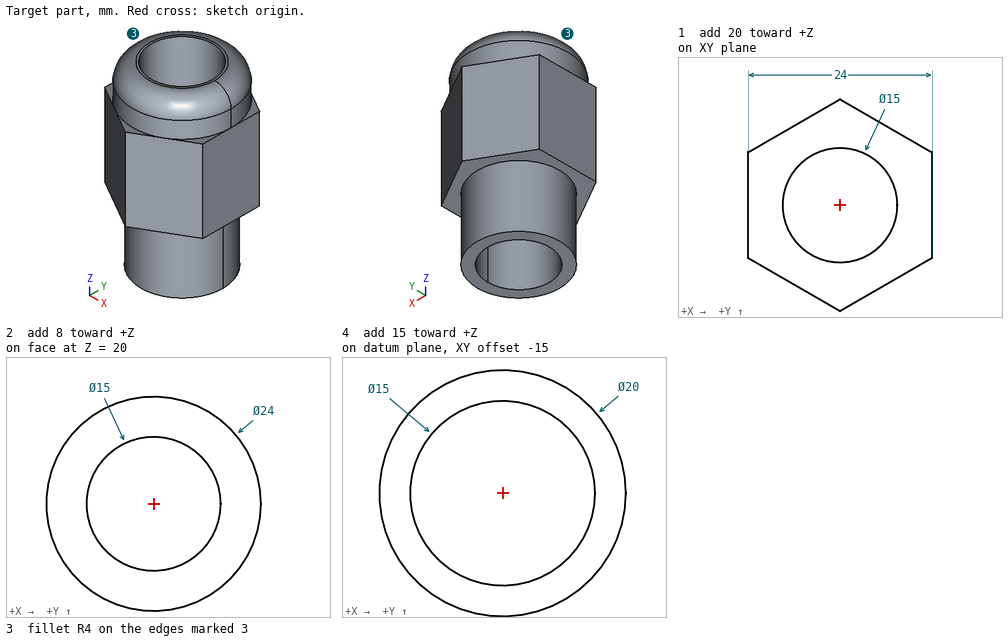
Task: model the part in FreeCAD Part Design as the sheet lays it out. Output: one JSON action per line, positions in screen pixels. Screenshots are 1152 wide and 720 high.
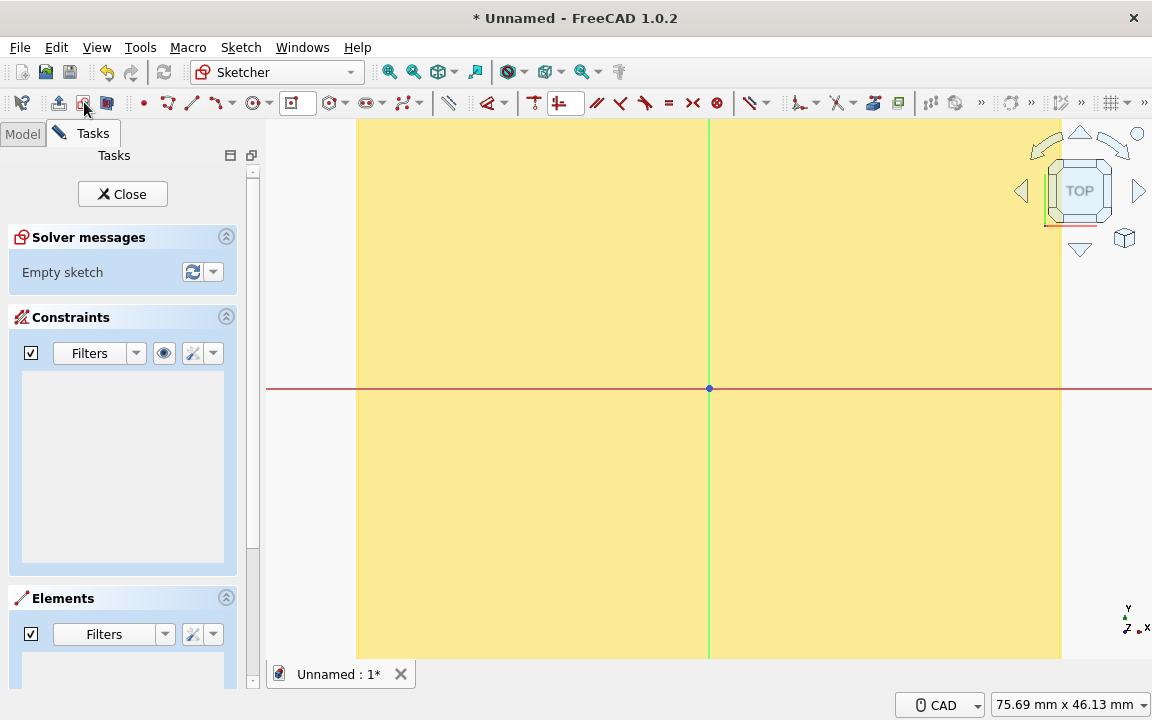
{"action": "scroll", "coordinate": [848, 389], "scroll_direction": "up", "scroll_amount": 2}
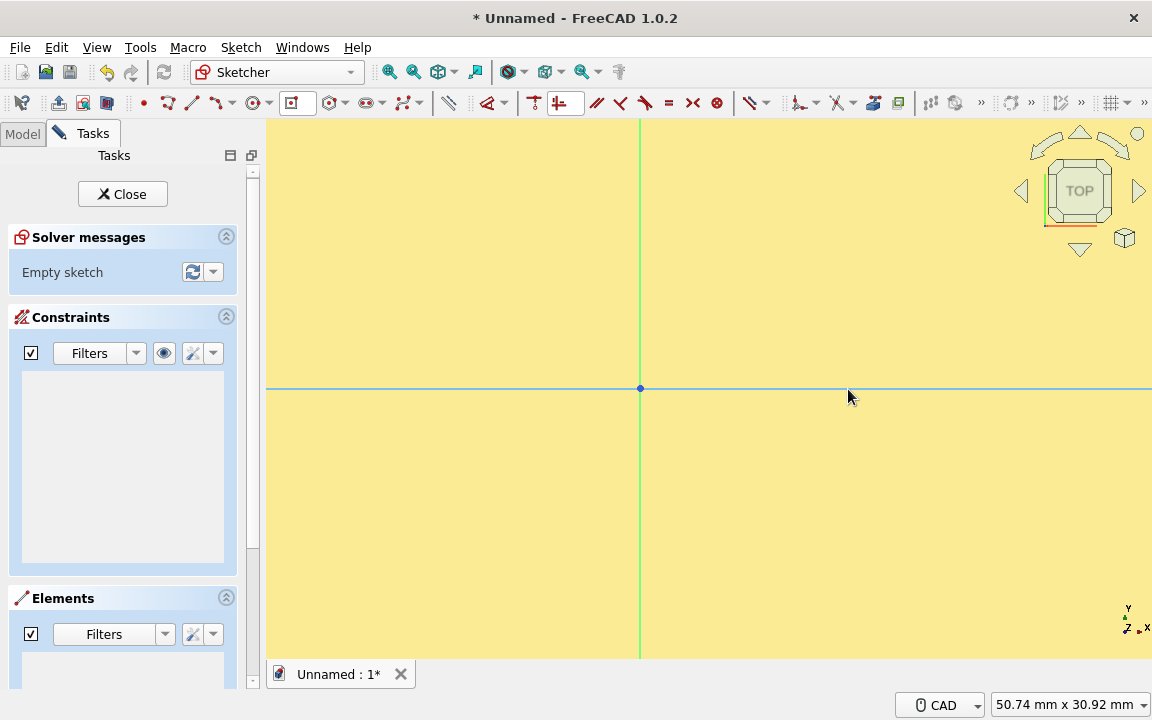
{"action": "key", "text": "g c"}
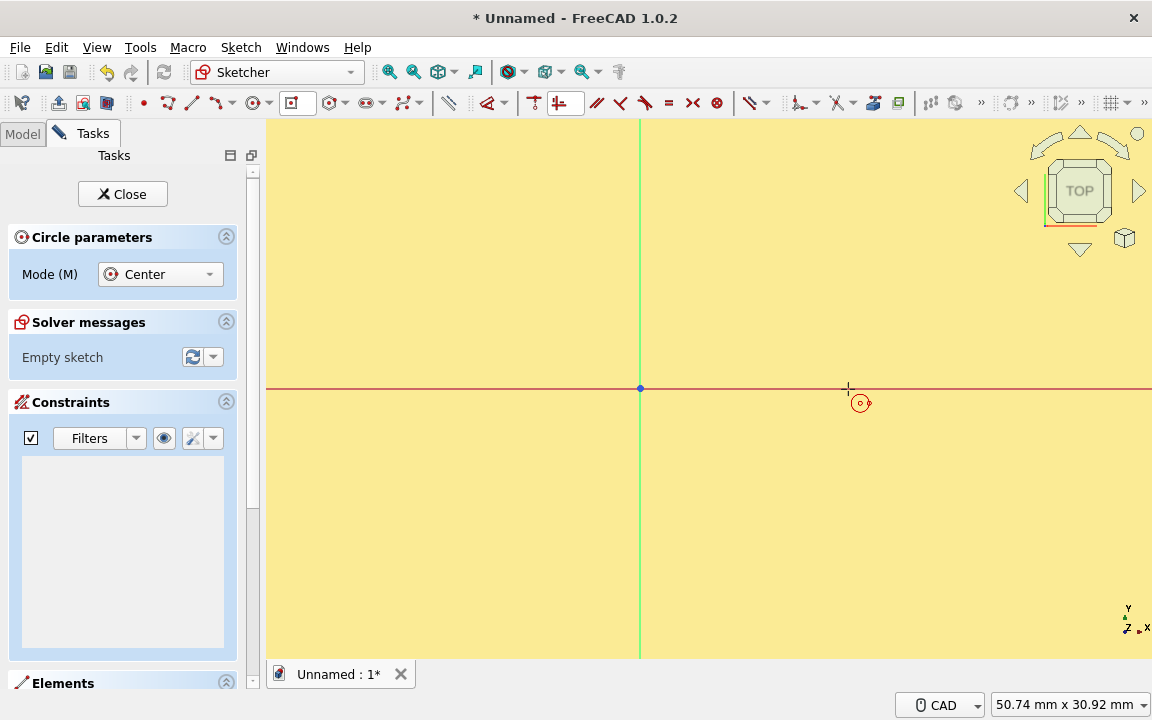
{"action": "left_click", "coordinate": [640, 389]}
{"action": "mouse_move", "coordinate": [764, 265]}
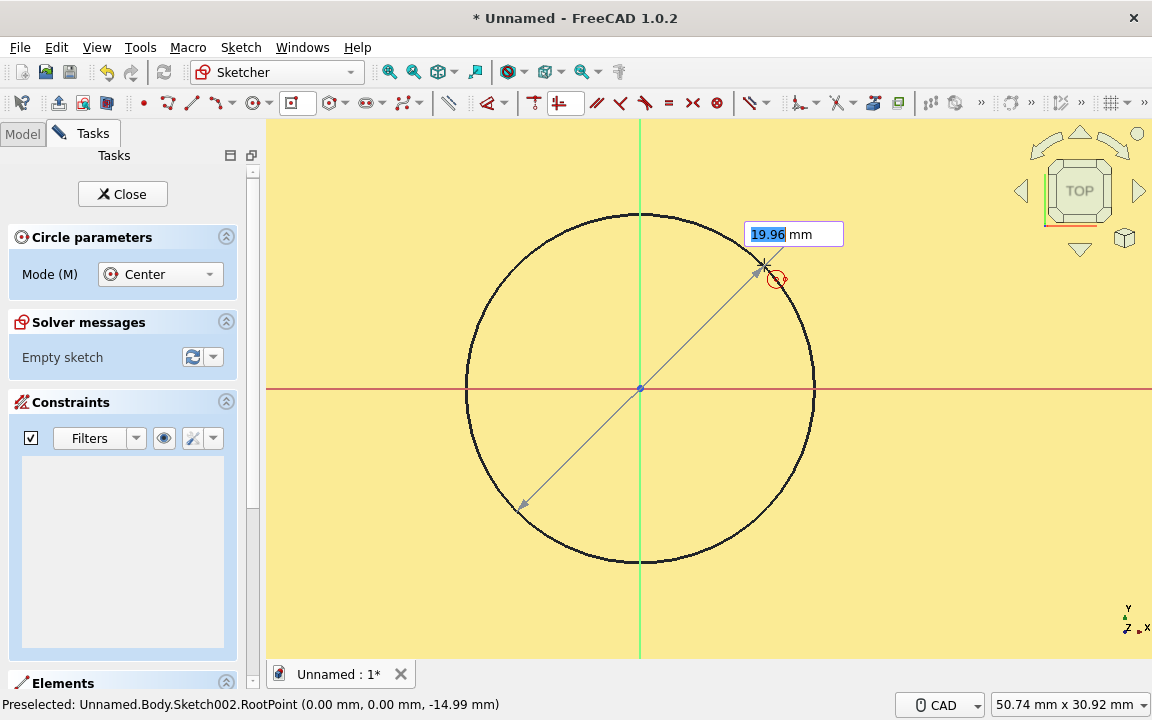
{"action": "type", "text": "20"}
{"action": "key", "text": "Return"}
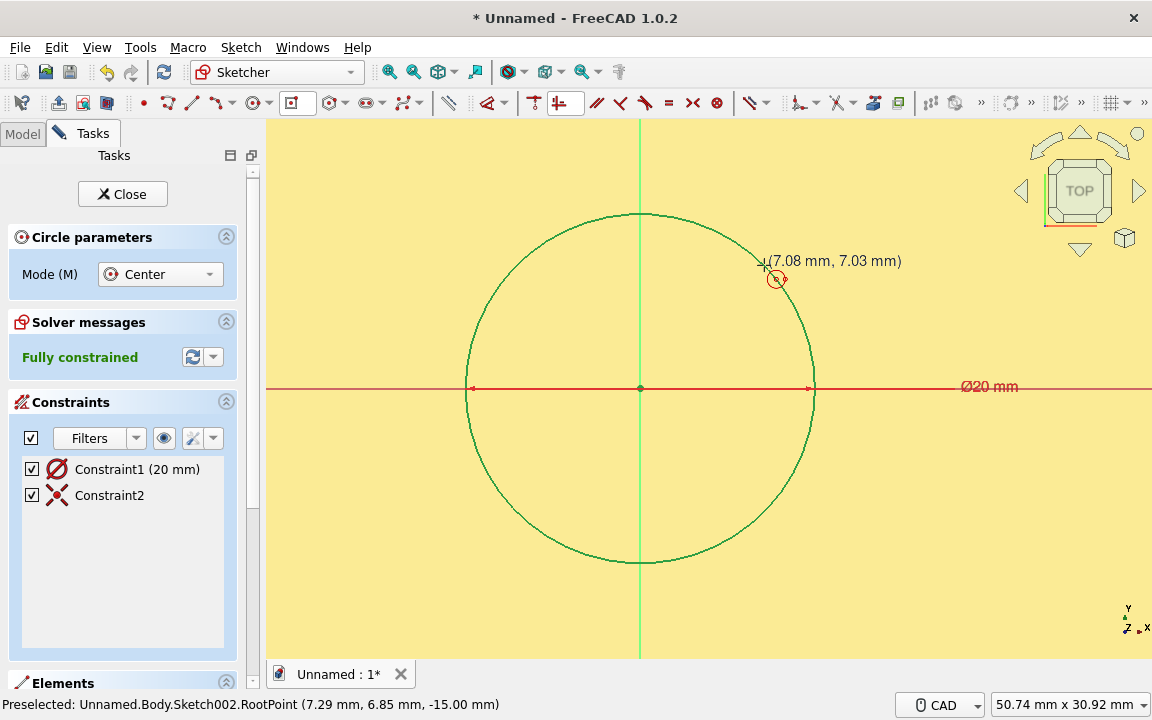
{"action": "left_click", "coordinate": [640, 389]}
{"action": "mouse_move", "coordinate": [733, 296]}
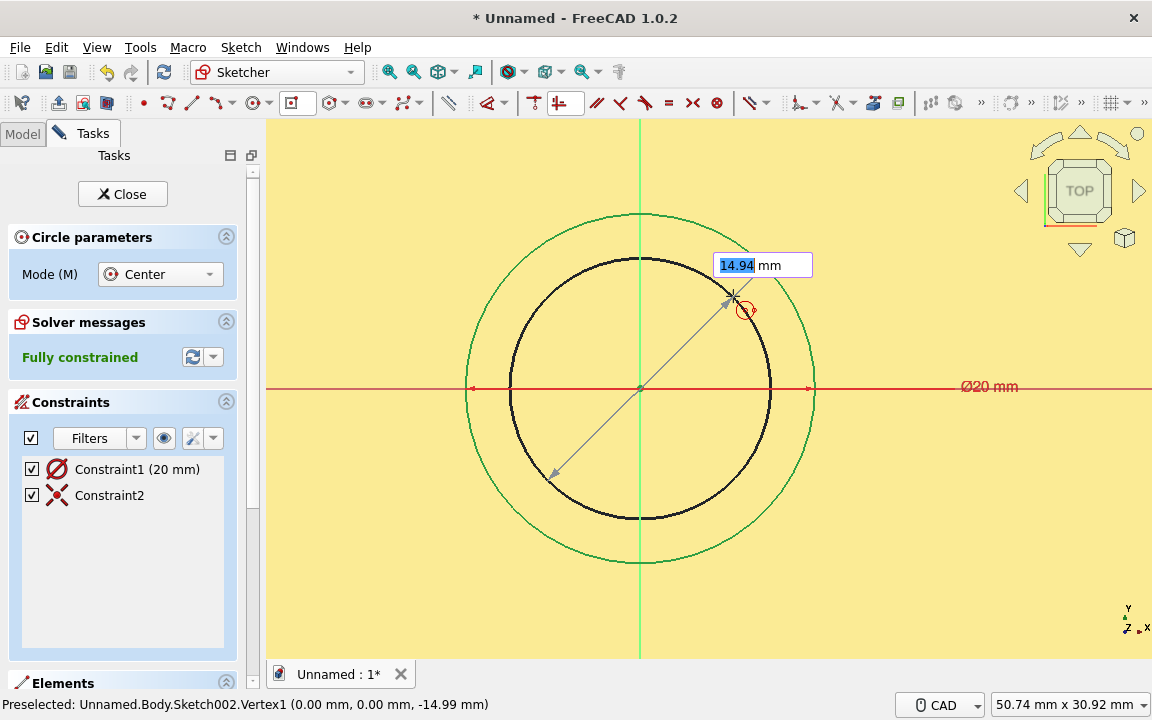
{"action": "type", "text": "15"}
{"action": "key", "text": "Return"}
{"action": "key", "text": "Escape"}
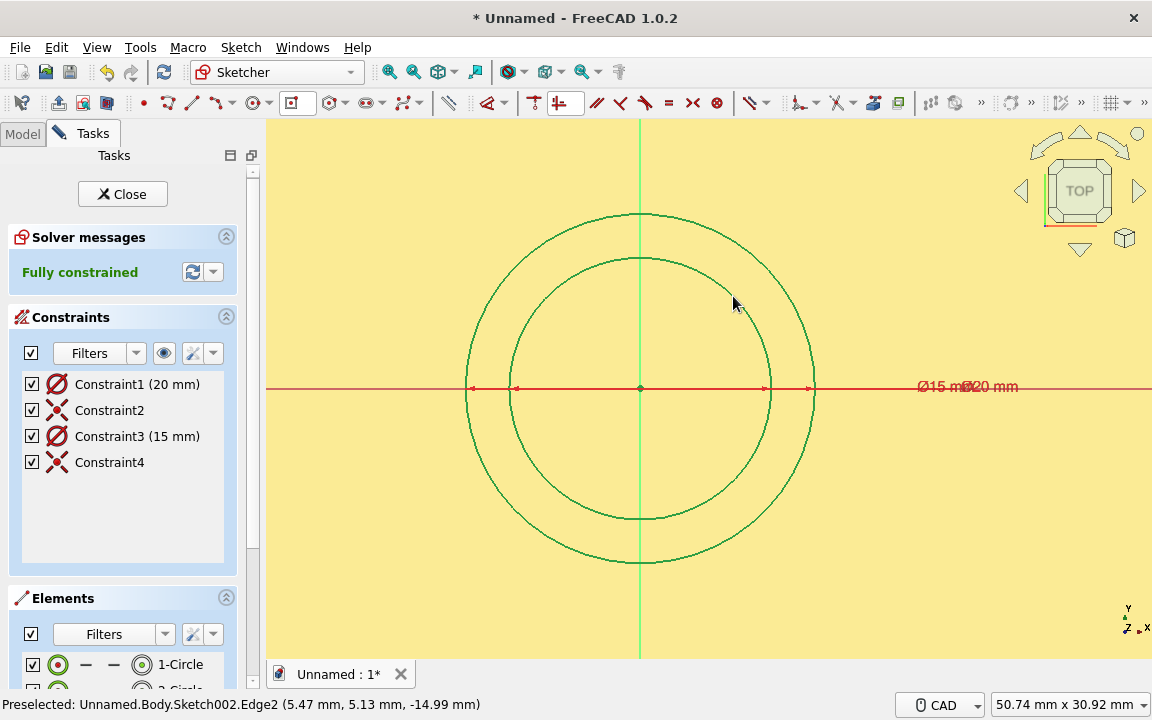
{"action": "left_click", "coordinate": [123, 194]}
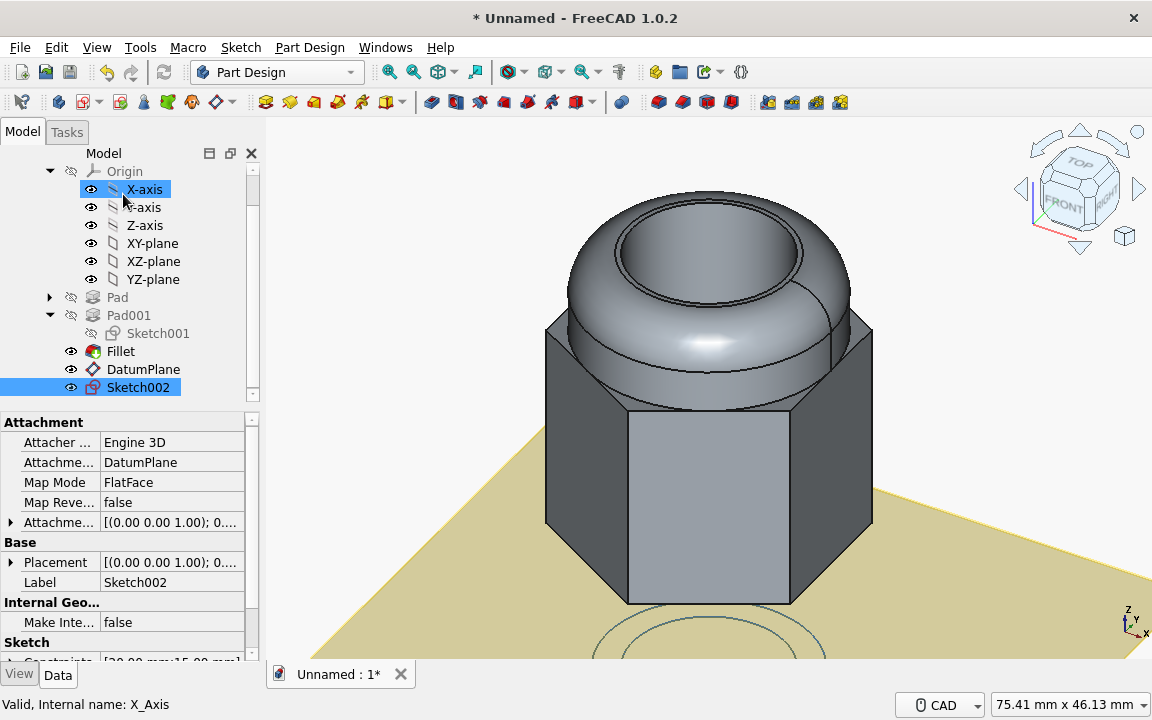
{"action": "left_click", "coordinate": [266, 102]}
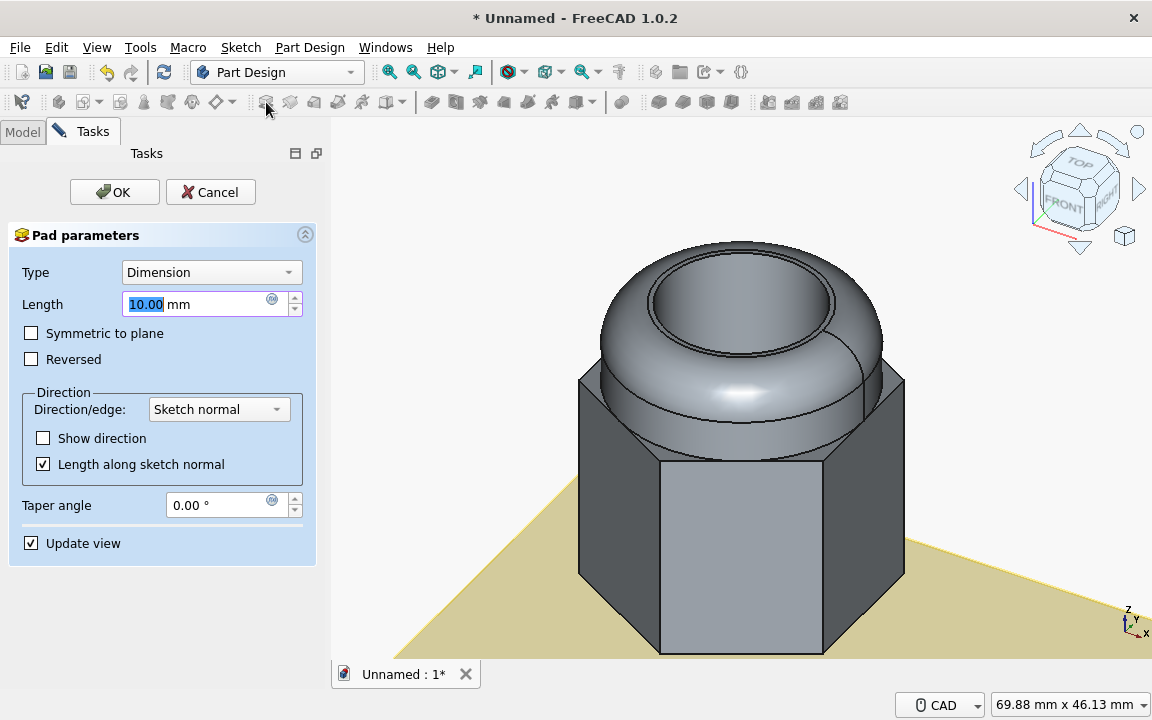
{"action": "type", "text": "15"}
{"action": "key", "text": "Tab"}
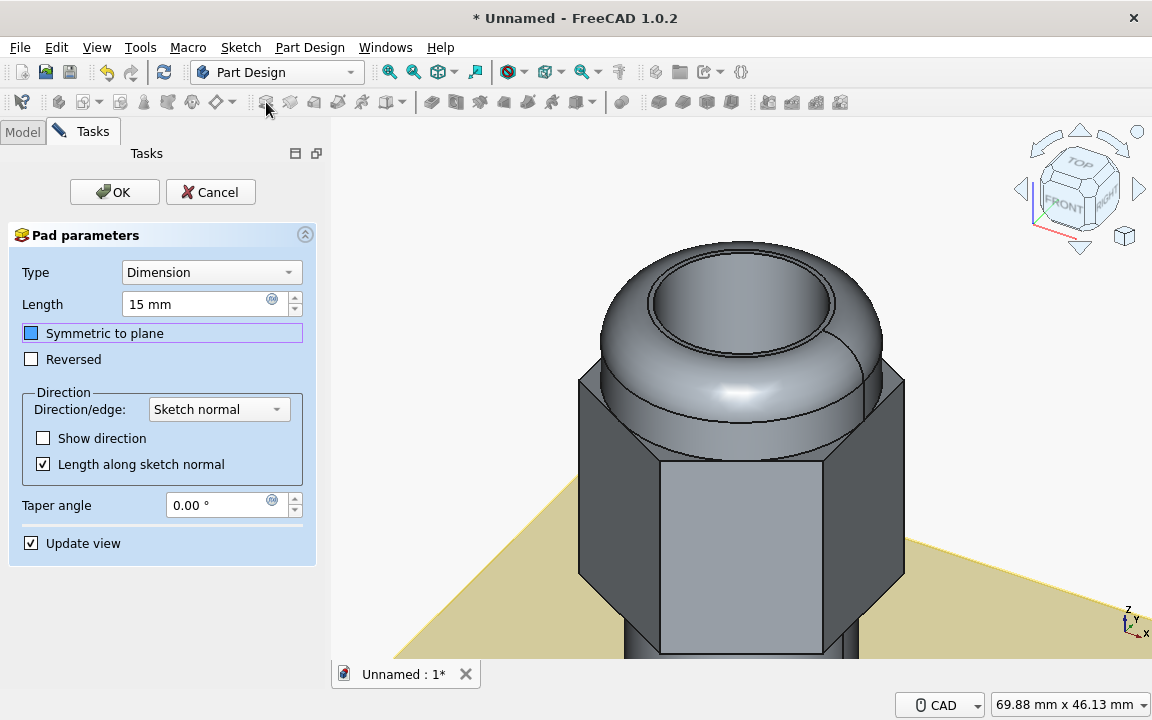
{"action": "left_click", "coordinate": [115, 192]}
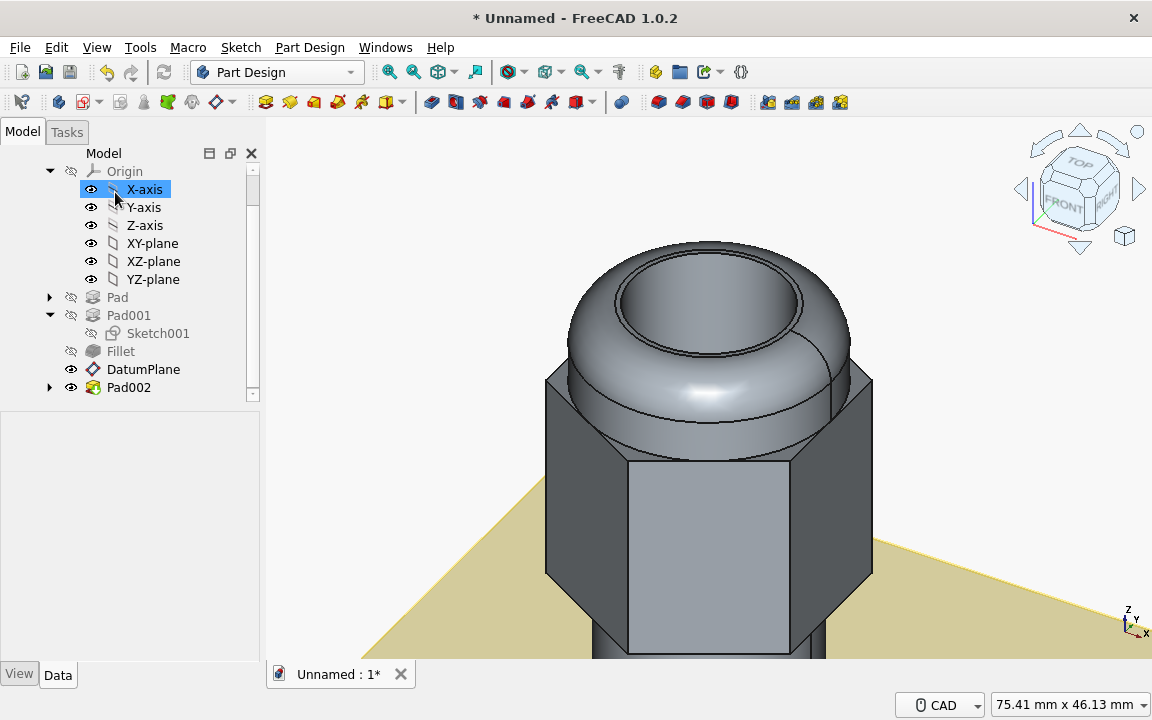
{"action": "left_click", "coordinate": [116, 369]}
{"action": "key", "text": "space"}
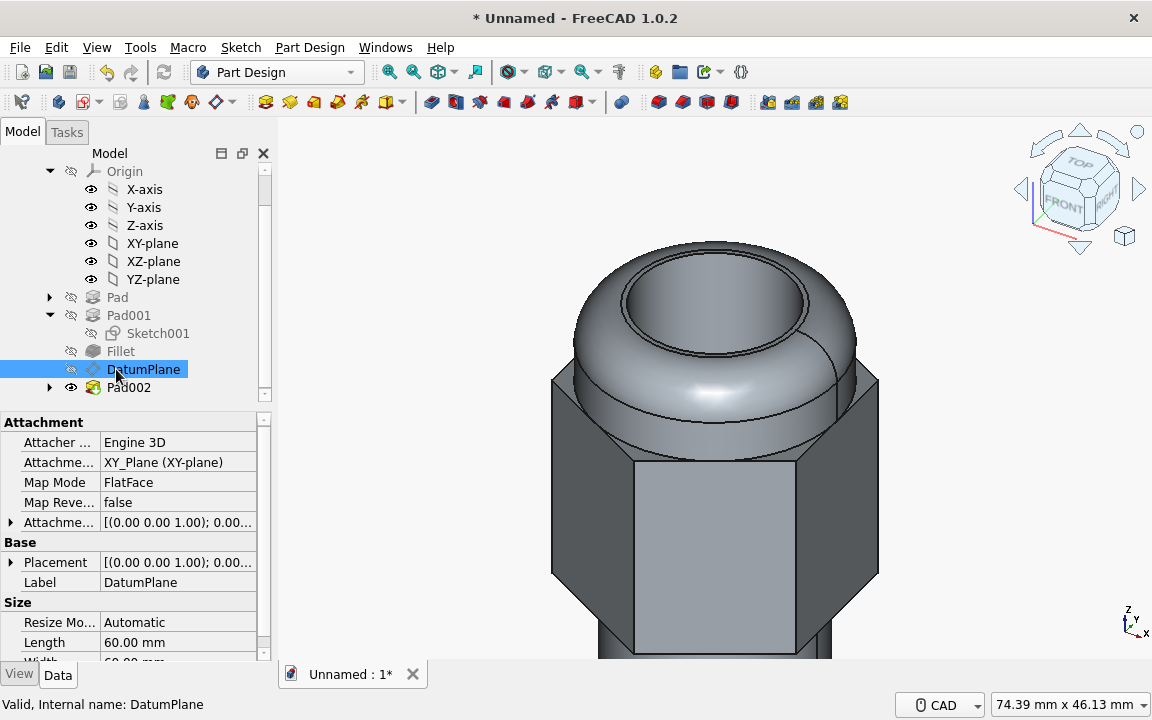
{"action": "key", "text": "0"}